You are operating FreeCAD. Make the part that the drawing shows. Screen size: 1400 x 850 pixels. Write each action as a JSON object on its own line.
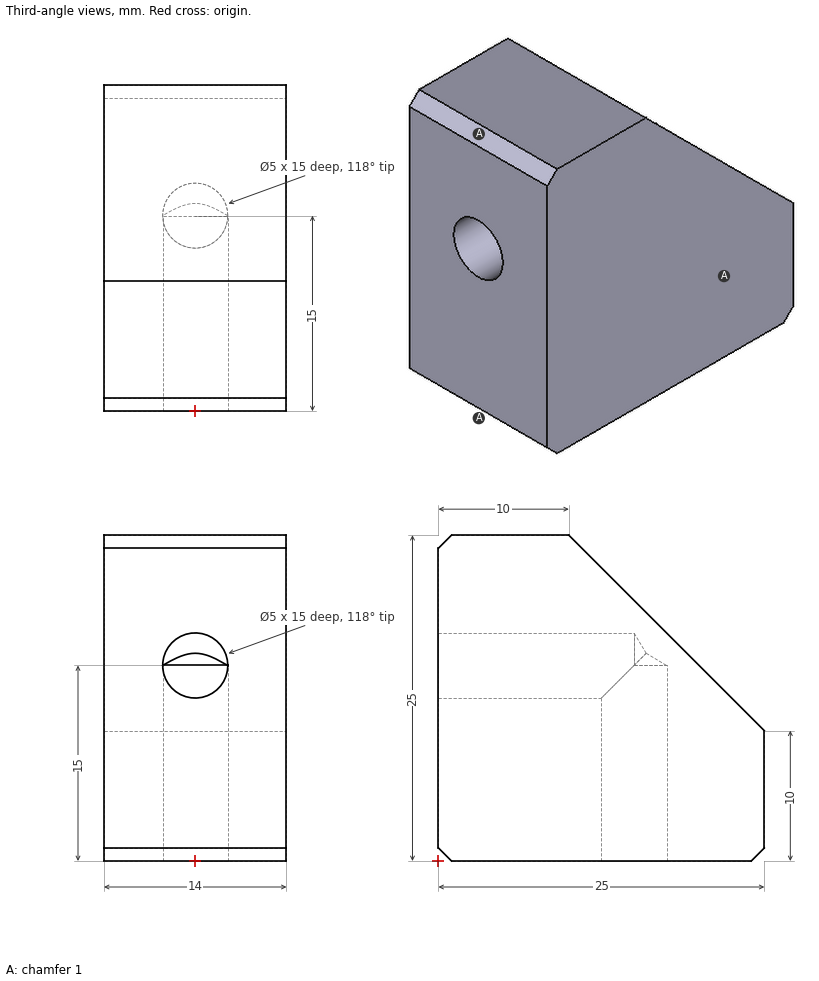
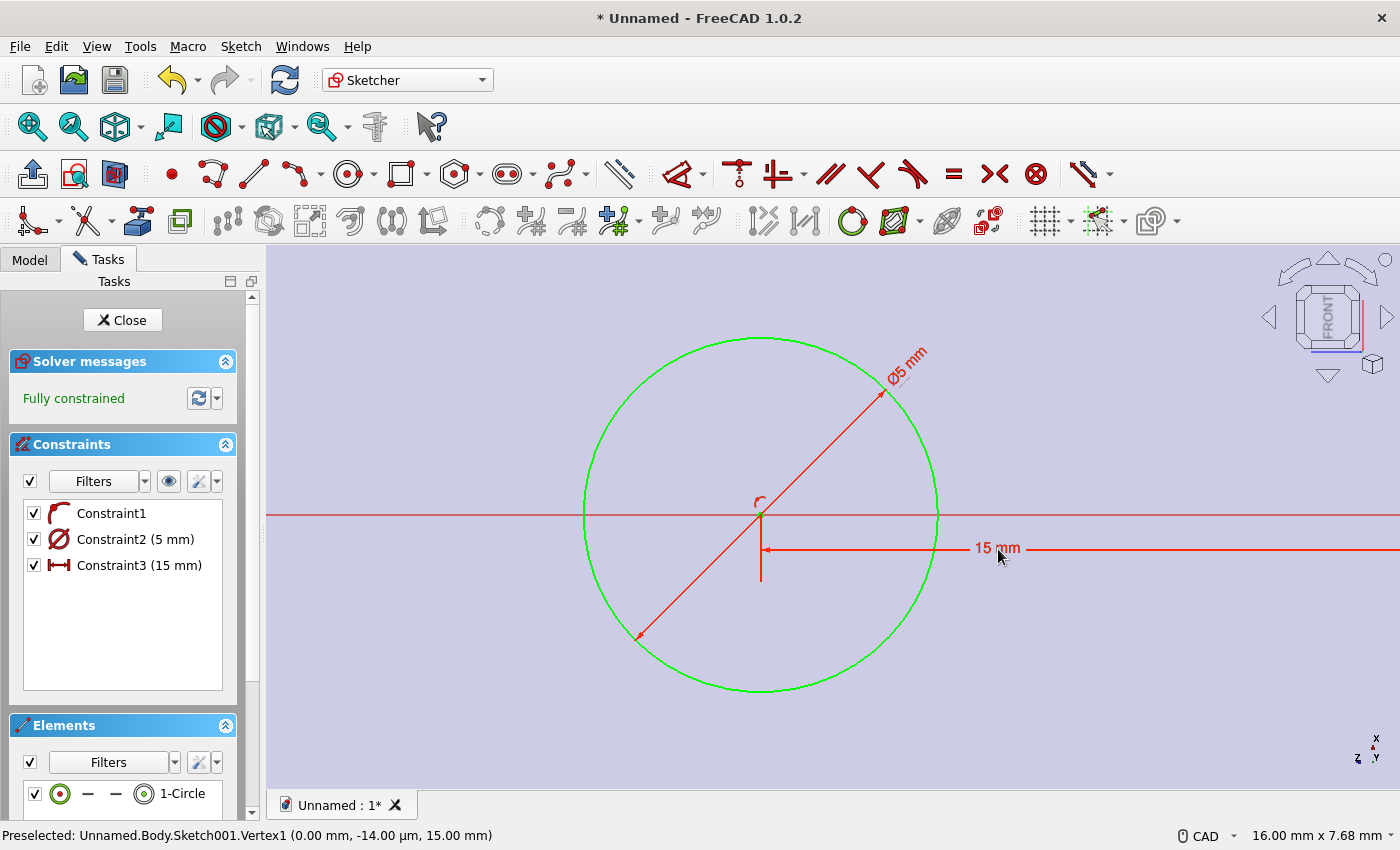
{"action": "left_click", "coordinate": [123, 320]}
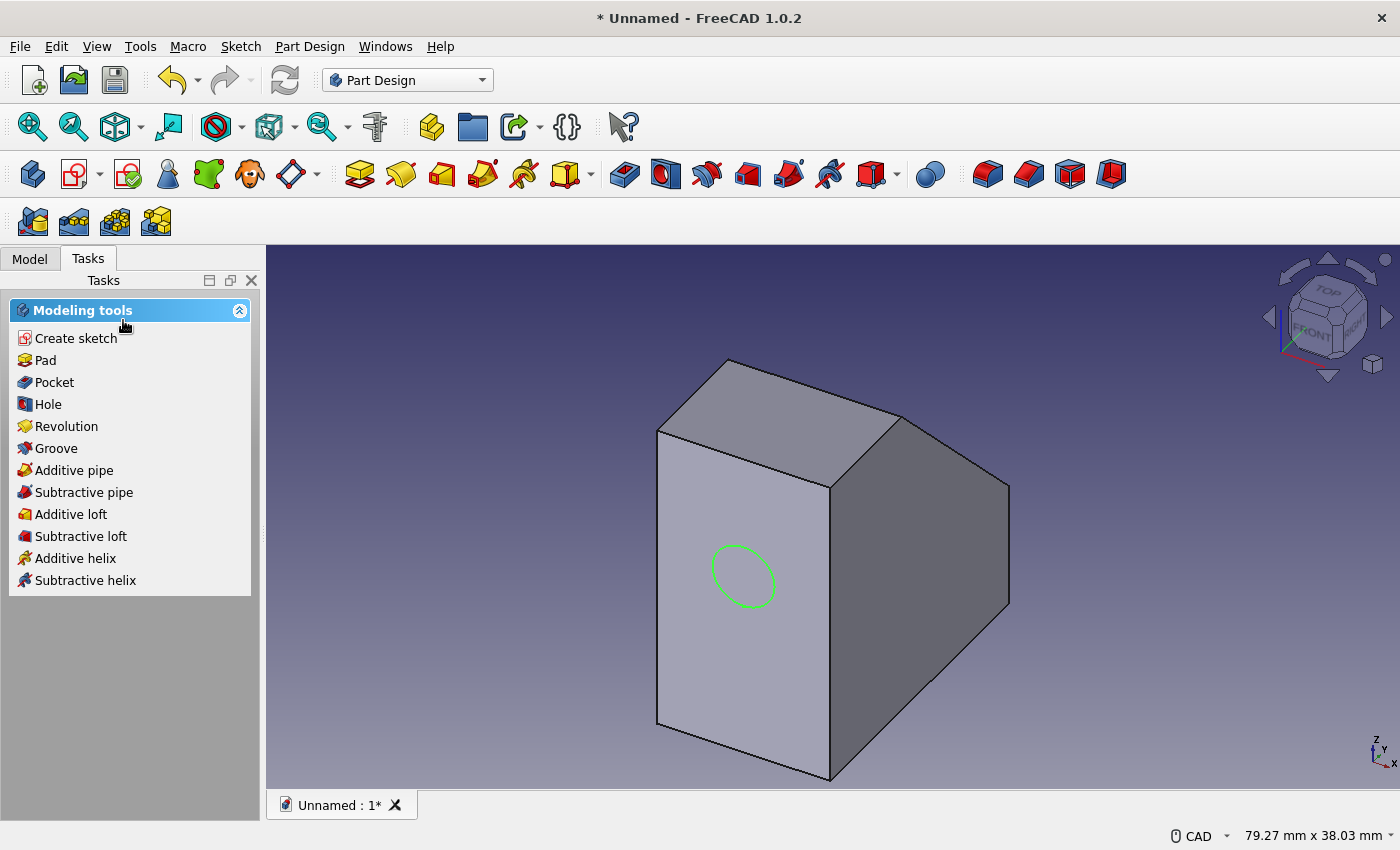
{"action": "left_click", "coordinate": [666, 174]}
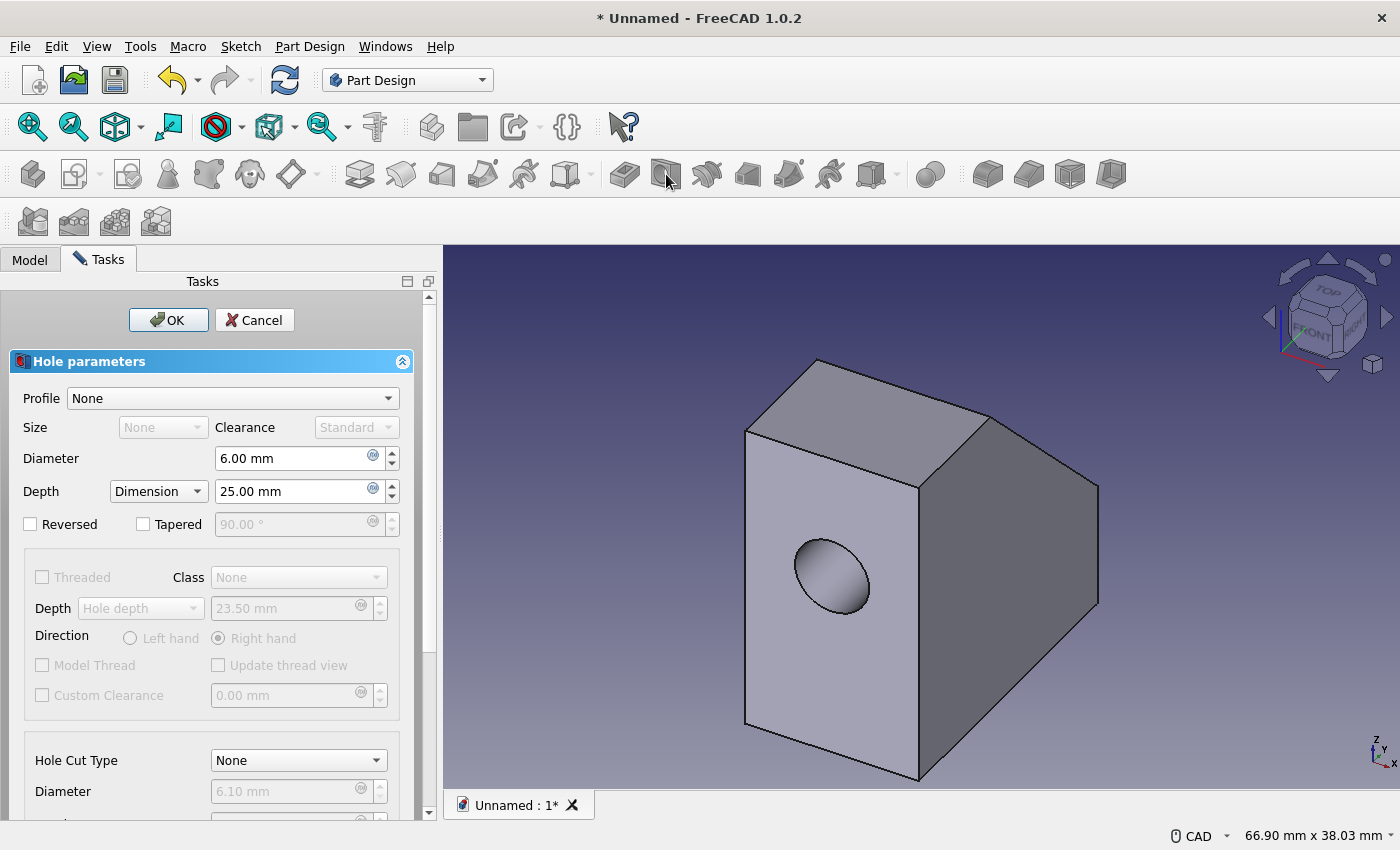
{"action": "triple_click", "coordinate": [300, 458]}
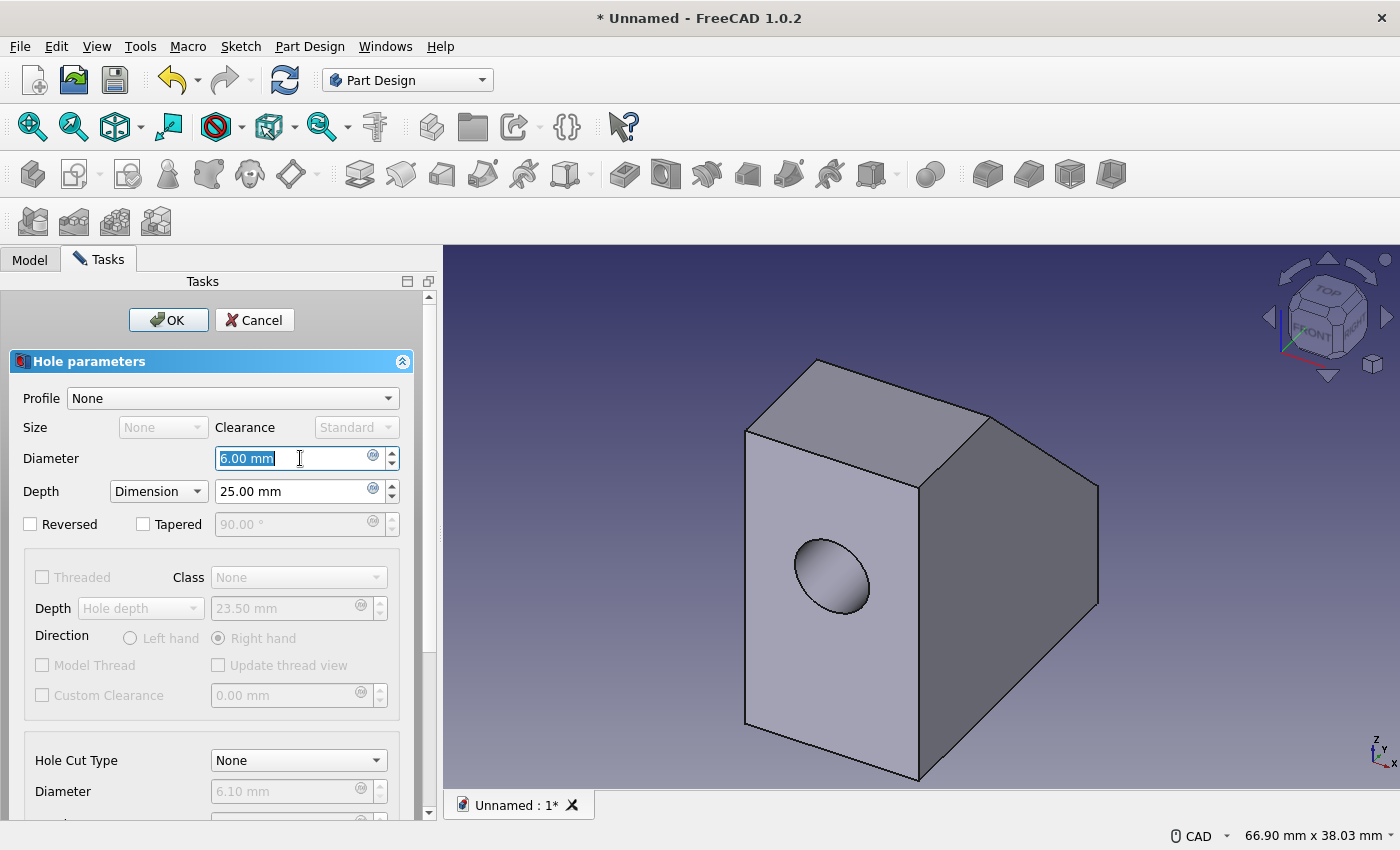
{"action": "type", "text": "5"}
{"action": "key", "text": "Tab"}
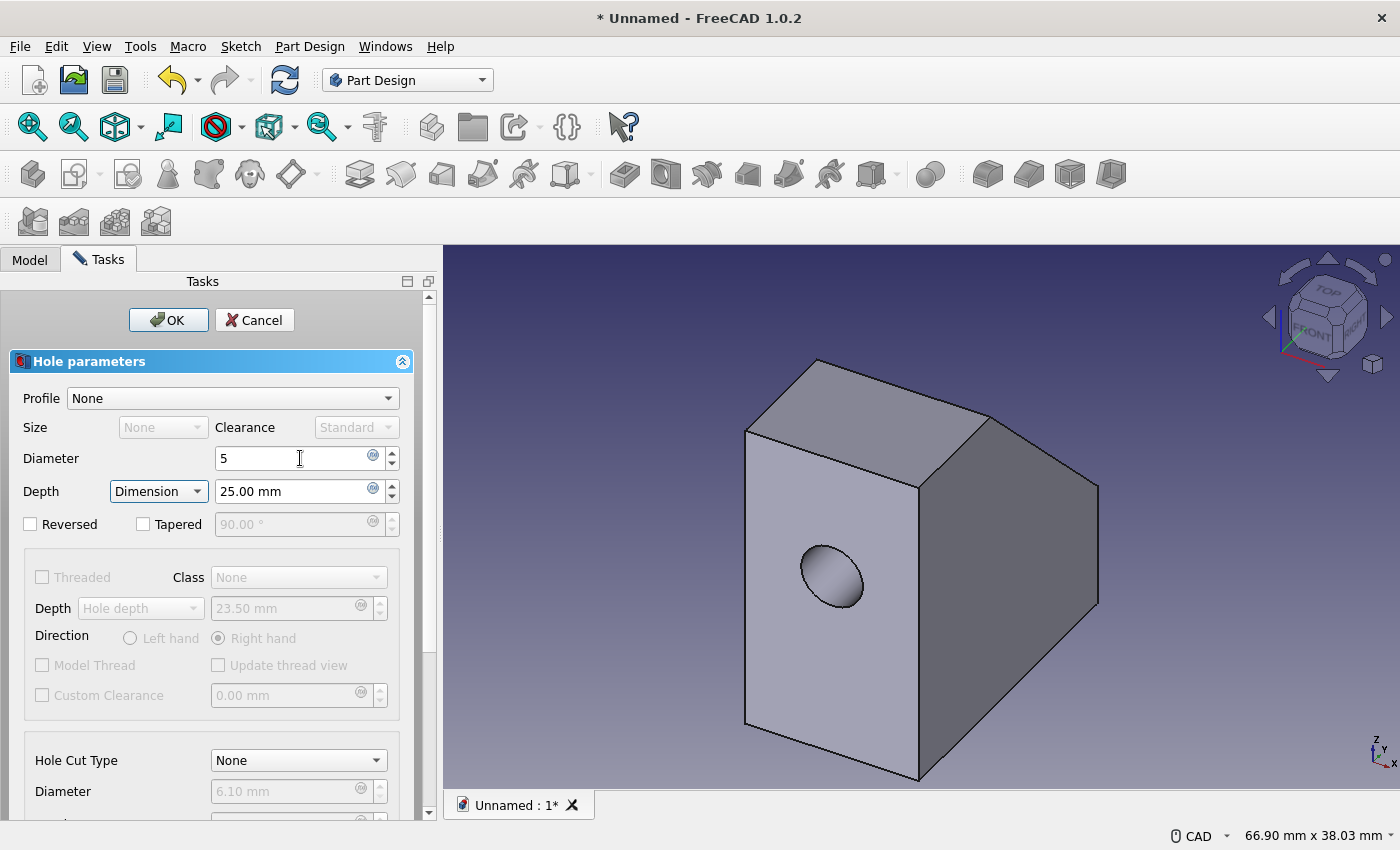
{"action": "triple_click", "coordinate": [300, 492]}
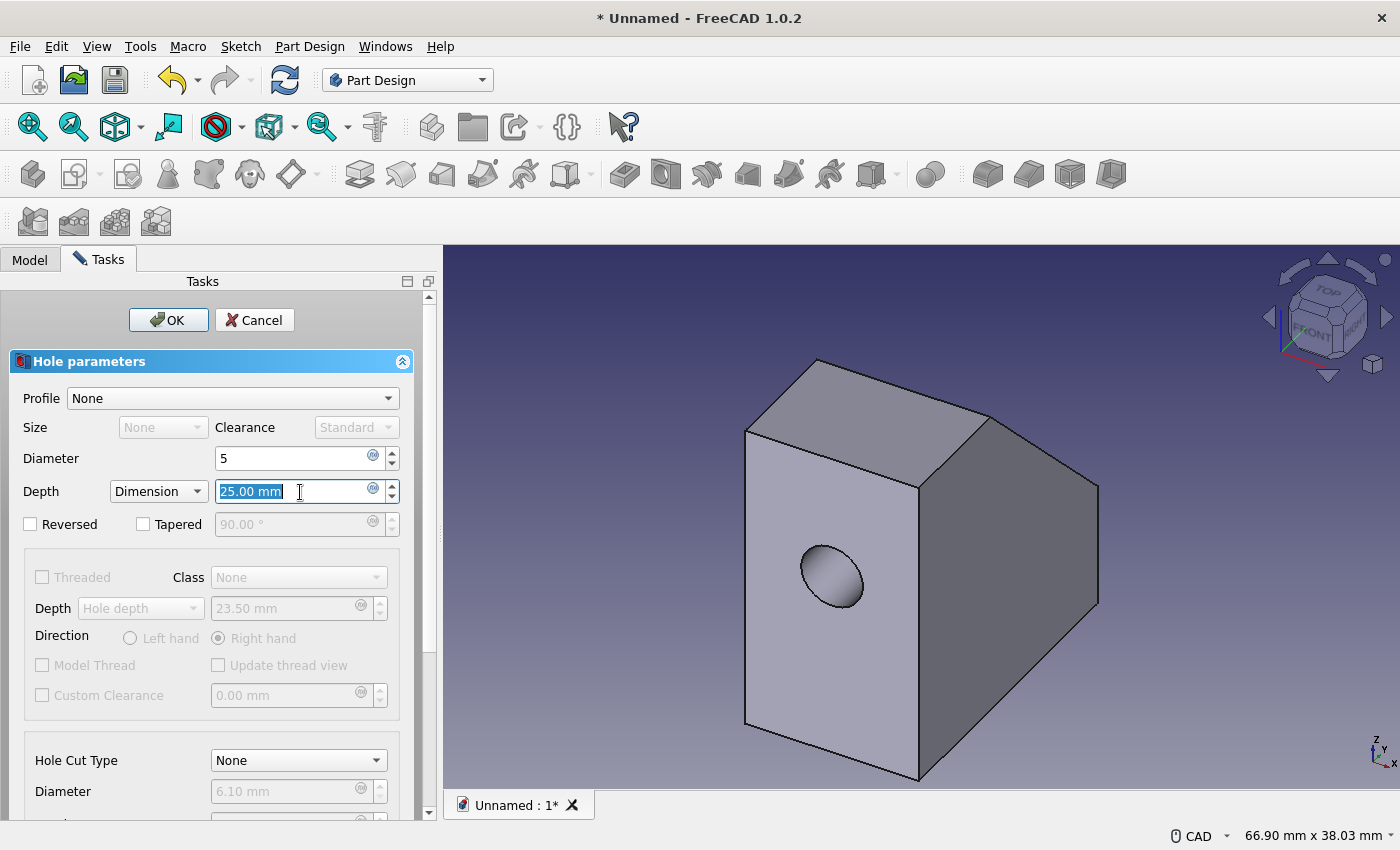
{"action": "type", "text": "15"}
{"action": "key", "text": "Tab"}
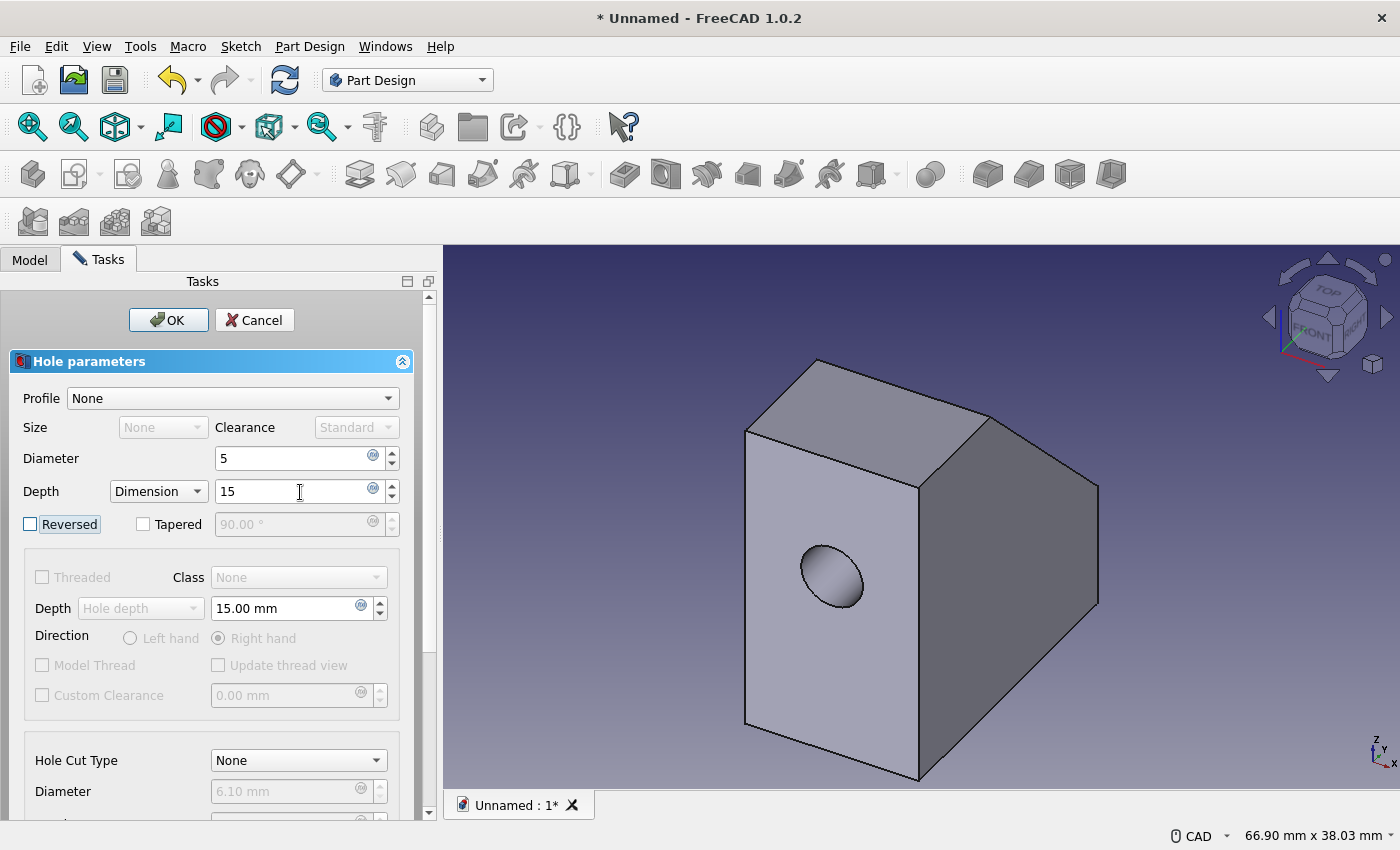
{"action": "left_click", "coordinate": [169, 320]}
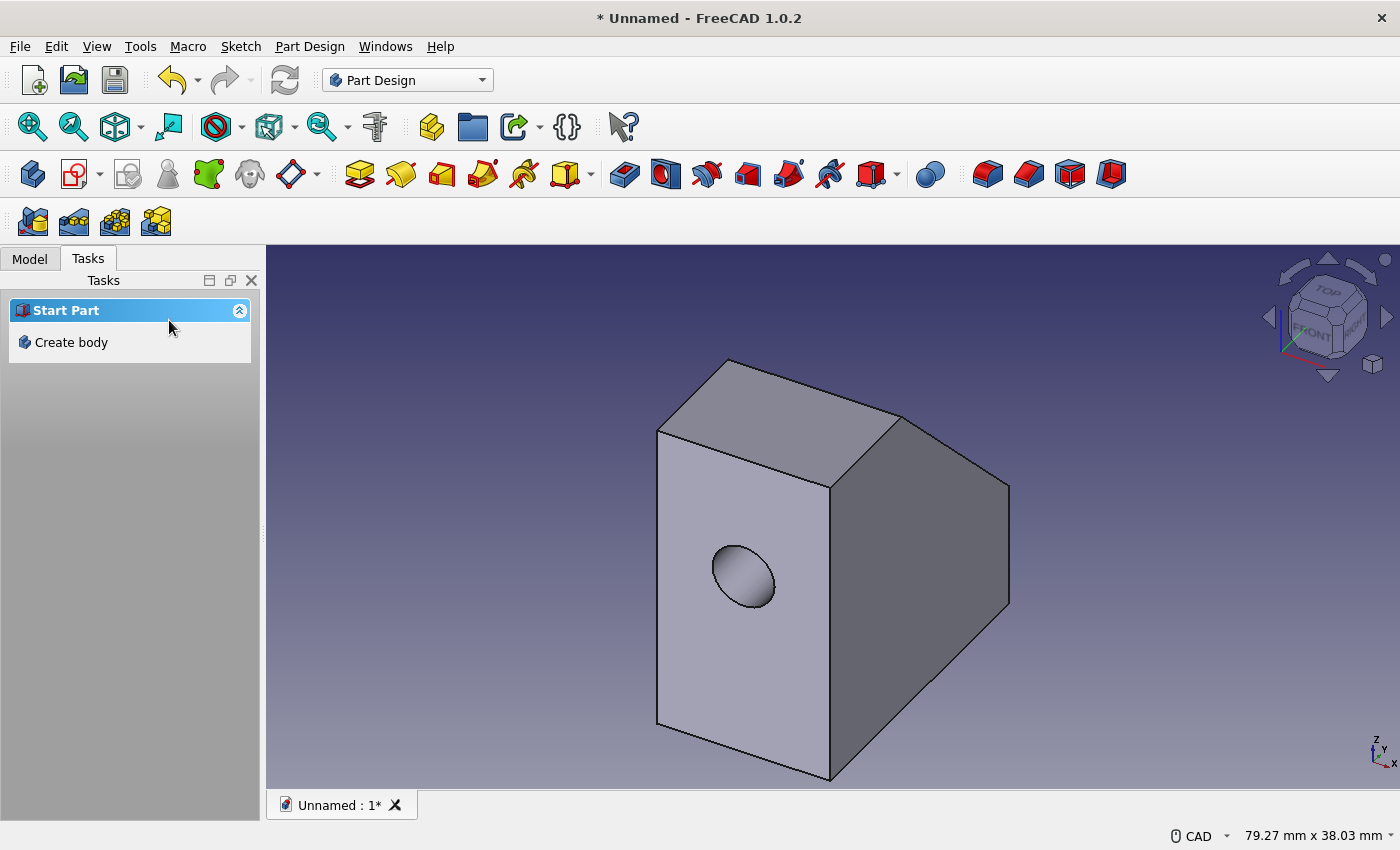
{"action": "left_click", "coordinate": [74, 174]}